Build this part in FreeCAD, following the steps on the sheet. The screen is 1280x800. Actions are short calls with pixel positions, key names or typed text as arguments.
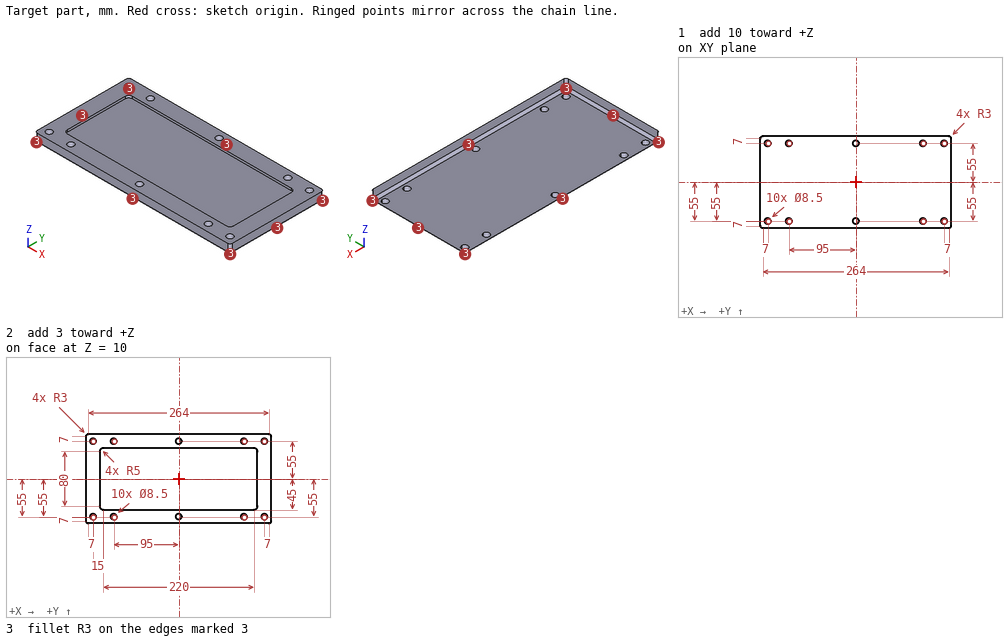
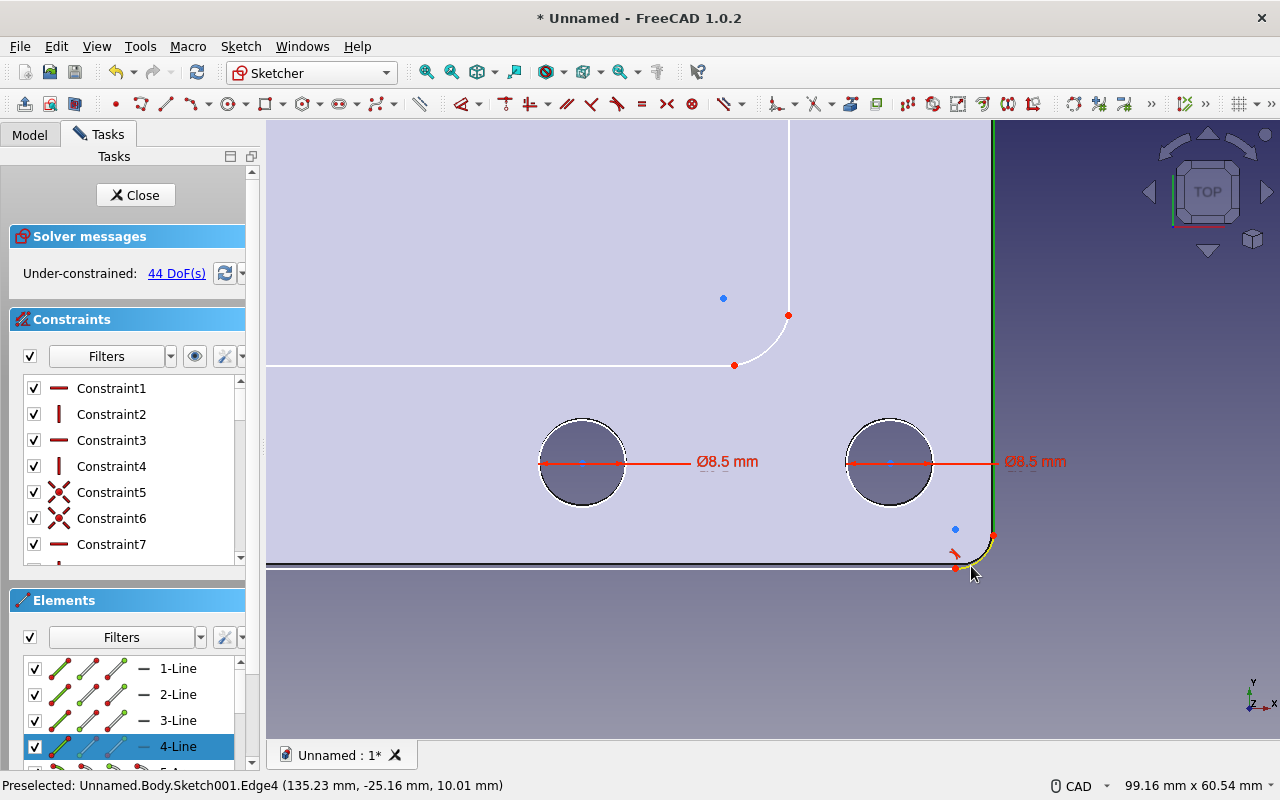
click(971, 565)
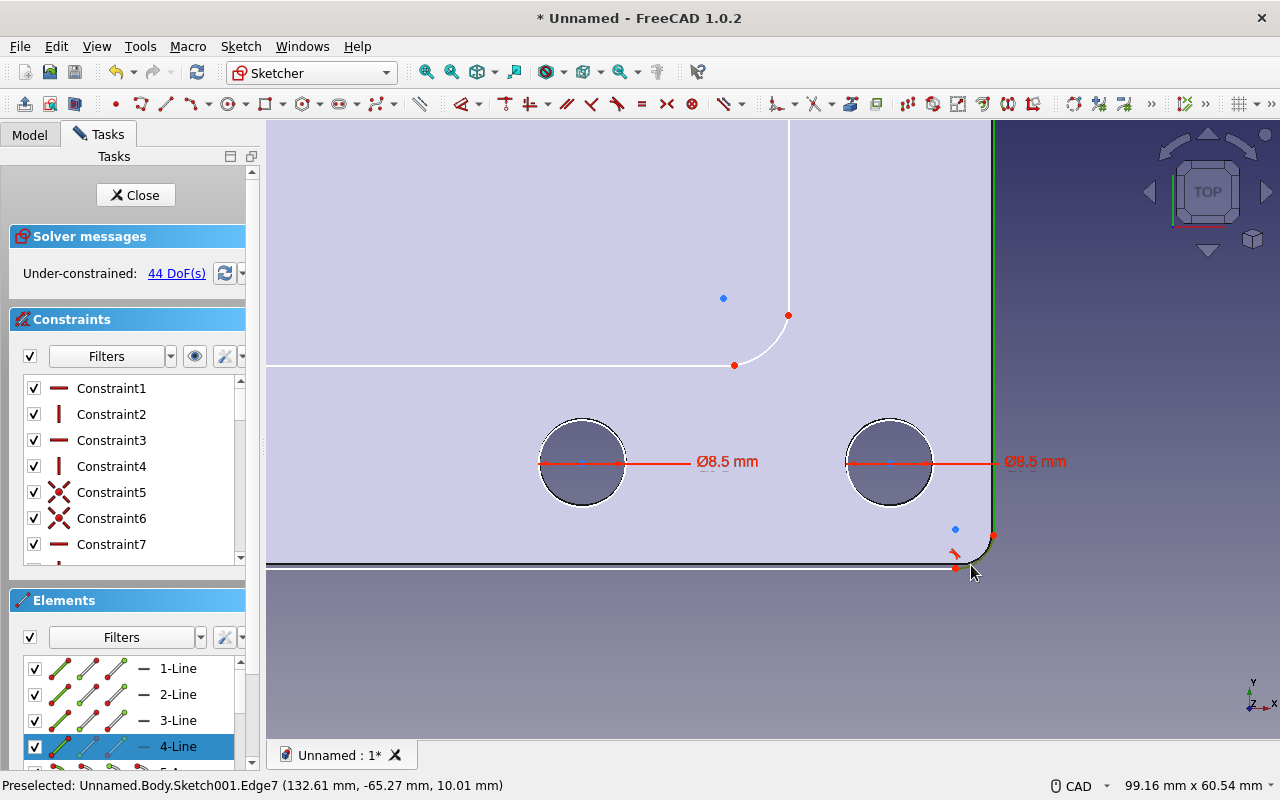
click(617, 104)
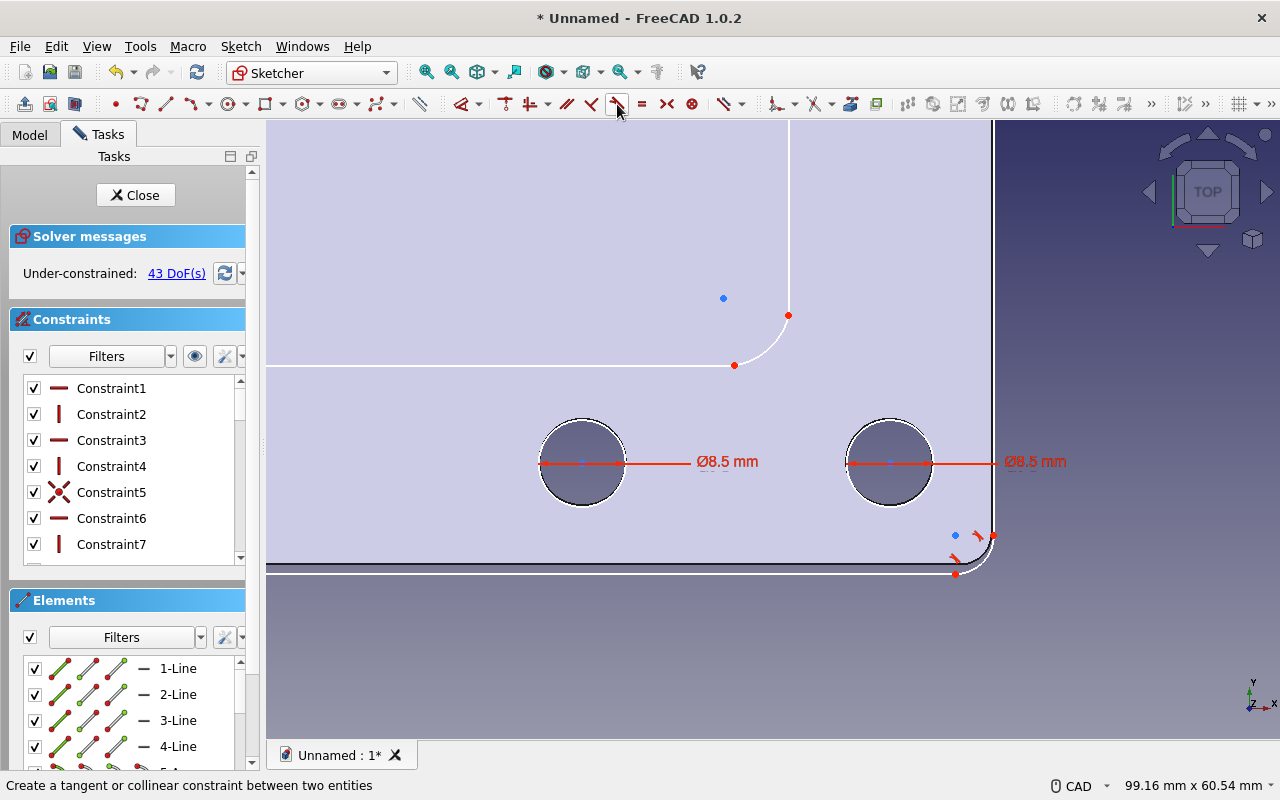
scroll(981, 564, down, 8)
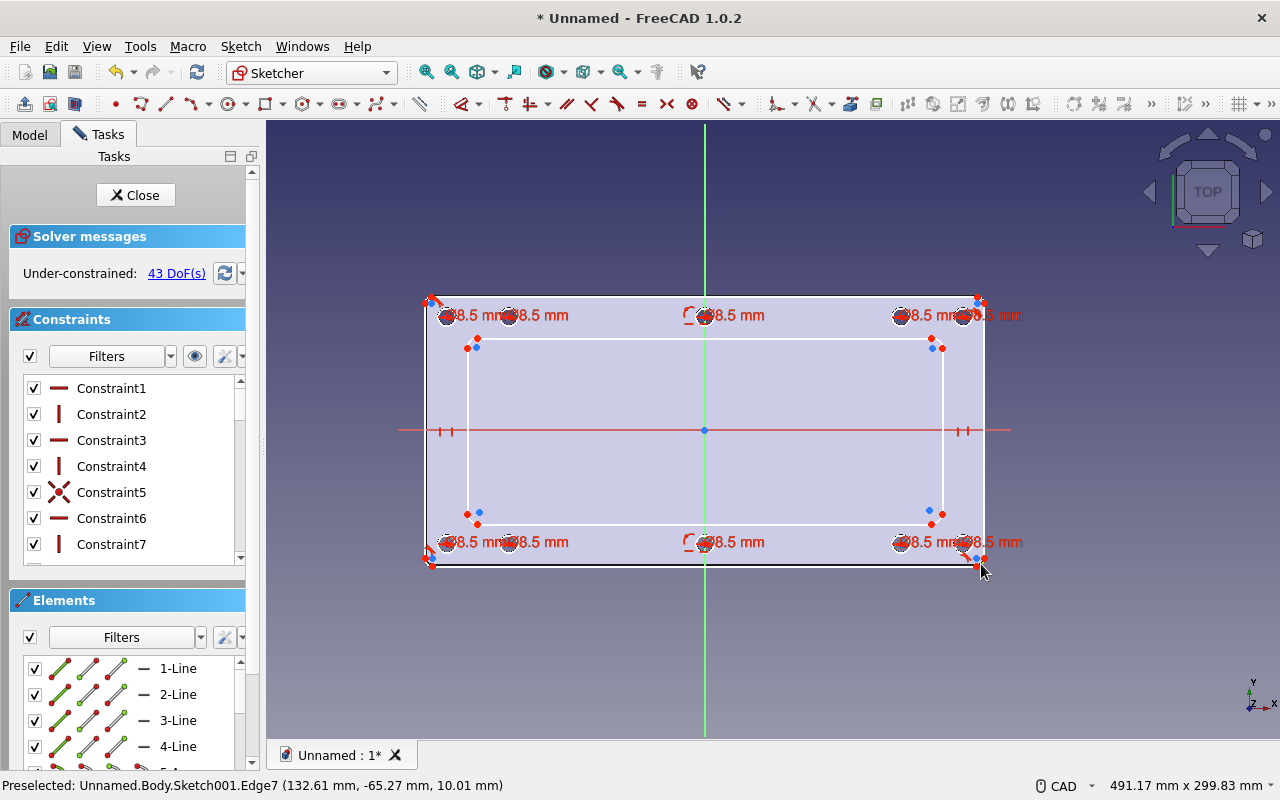
click(984, 482)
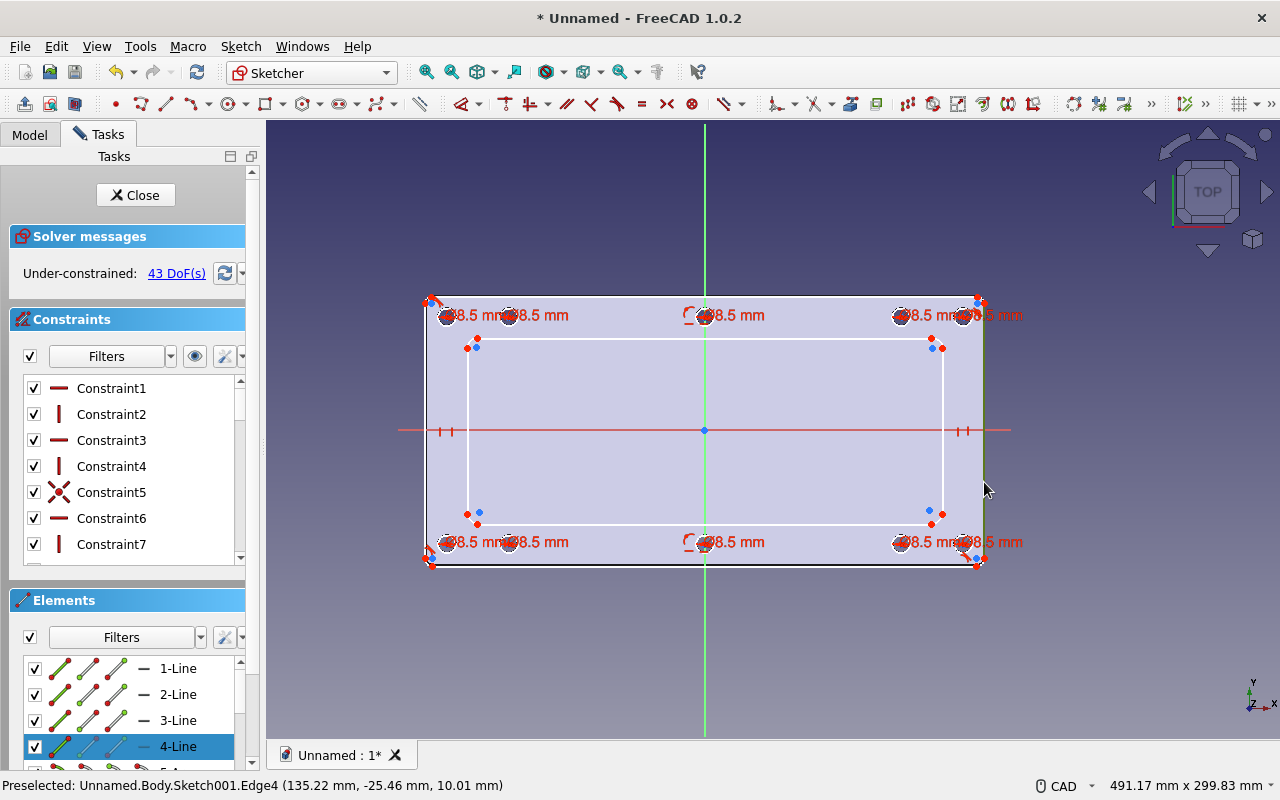
scroll(982, 299, up, 6)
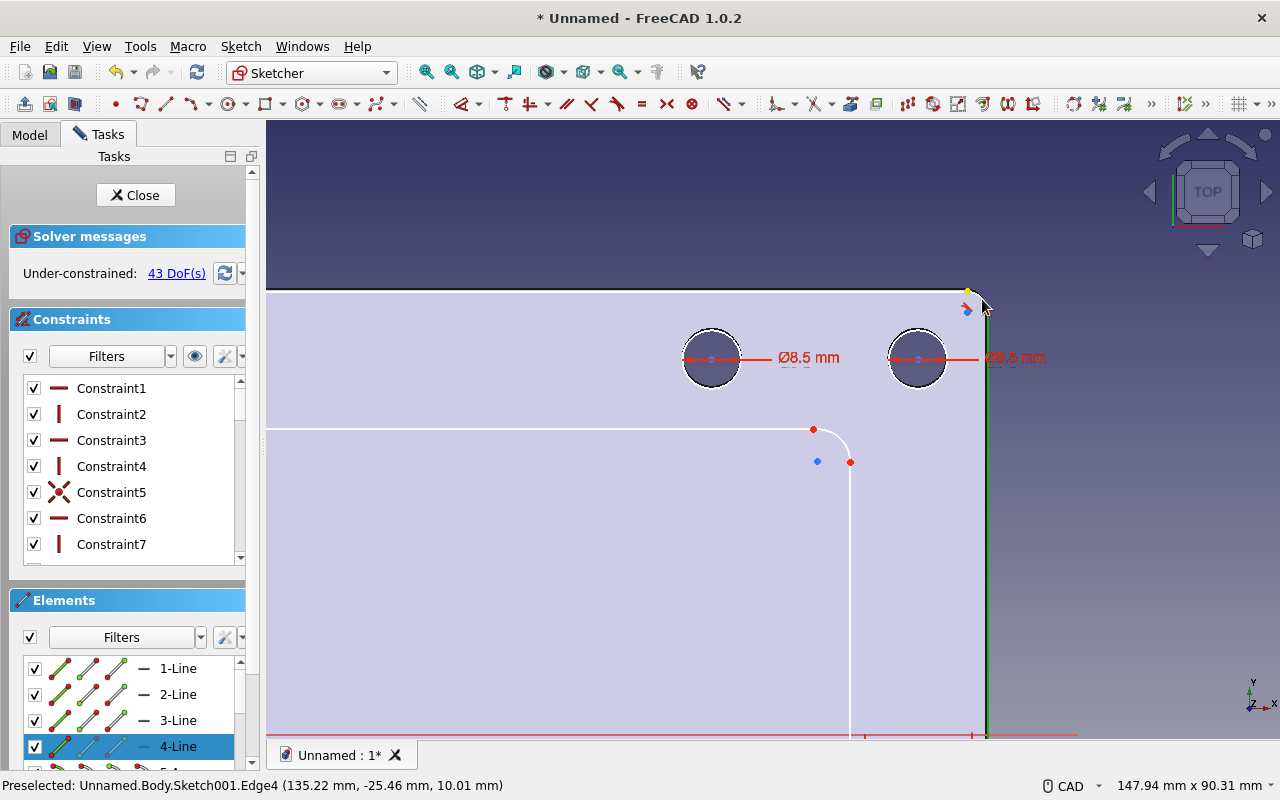
click(981, 298)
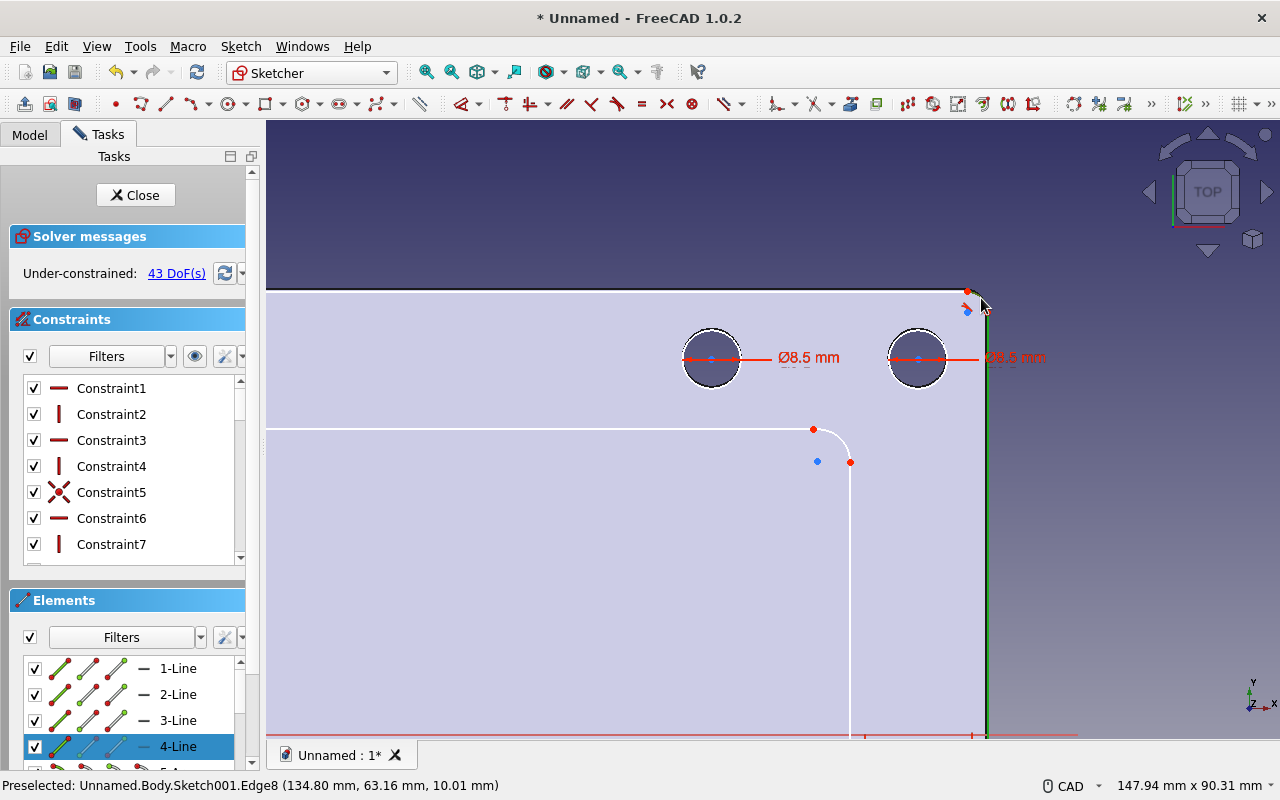
click(617, 104)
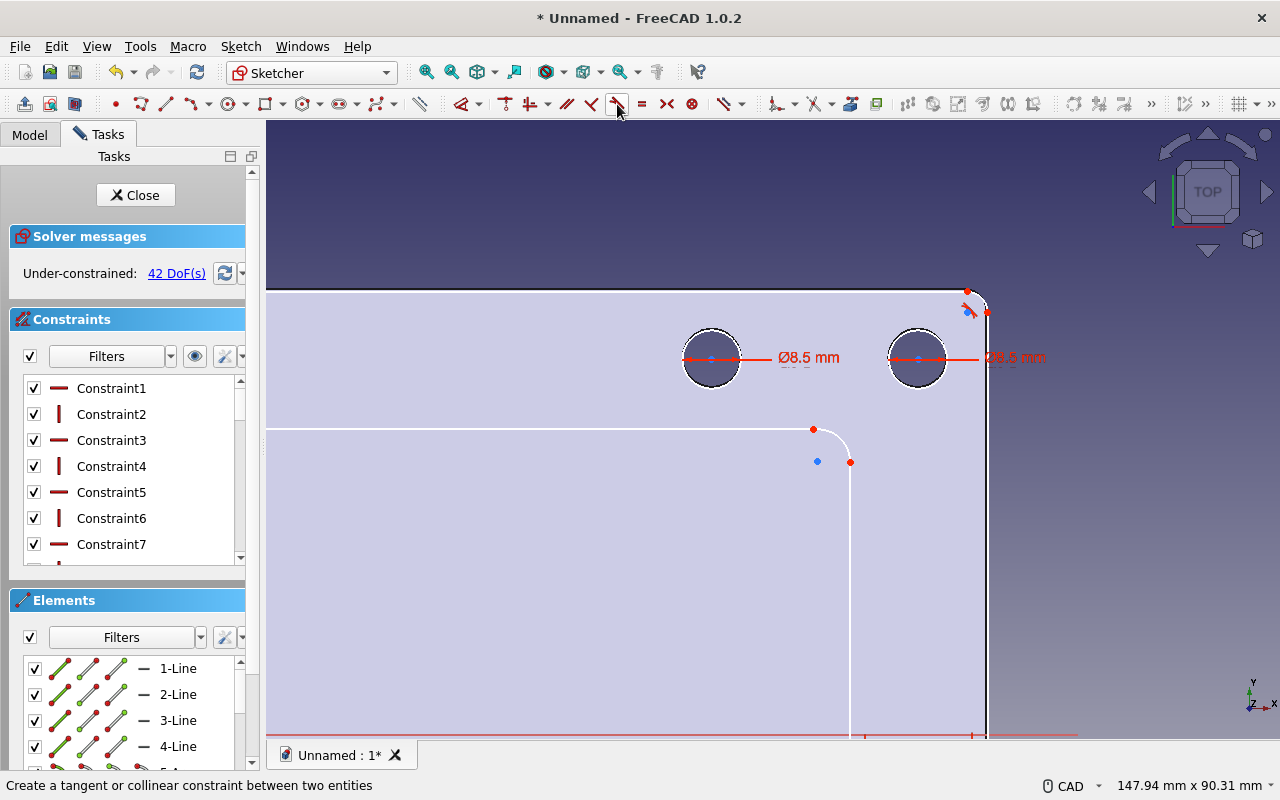
scroll(982, 298, down, 6)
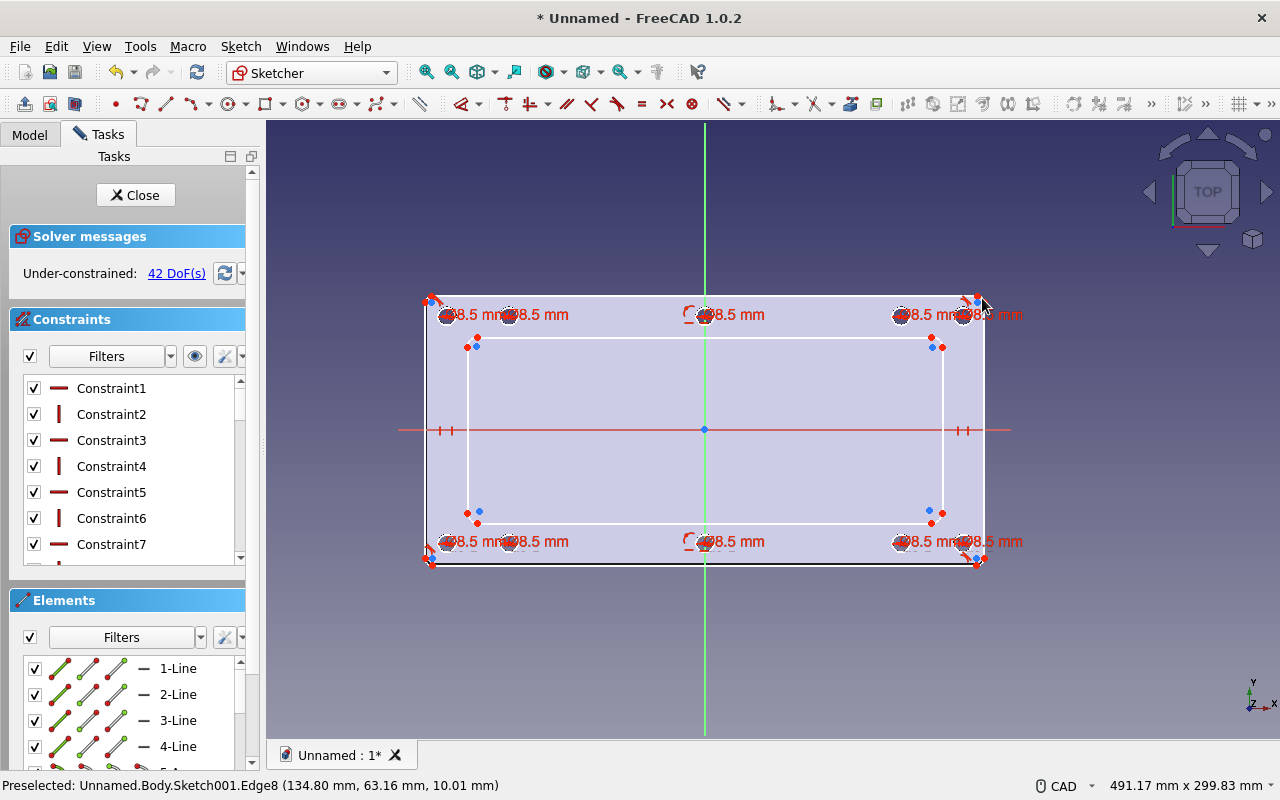
click(796, 524)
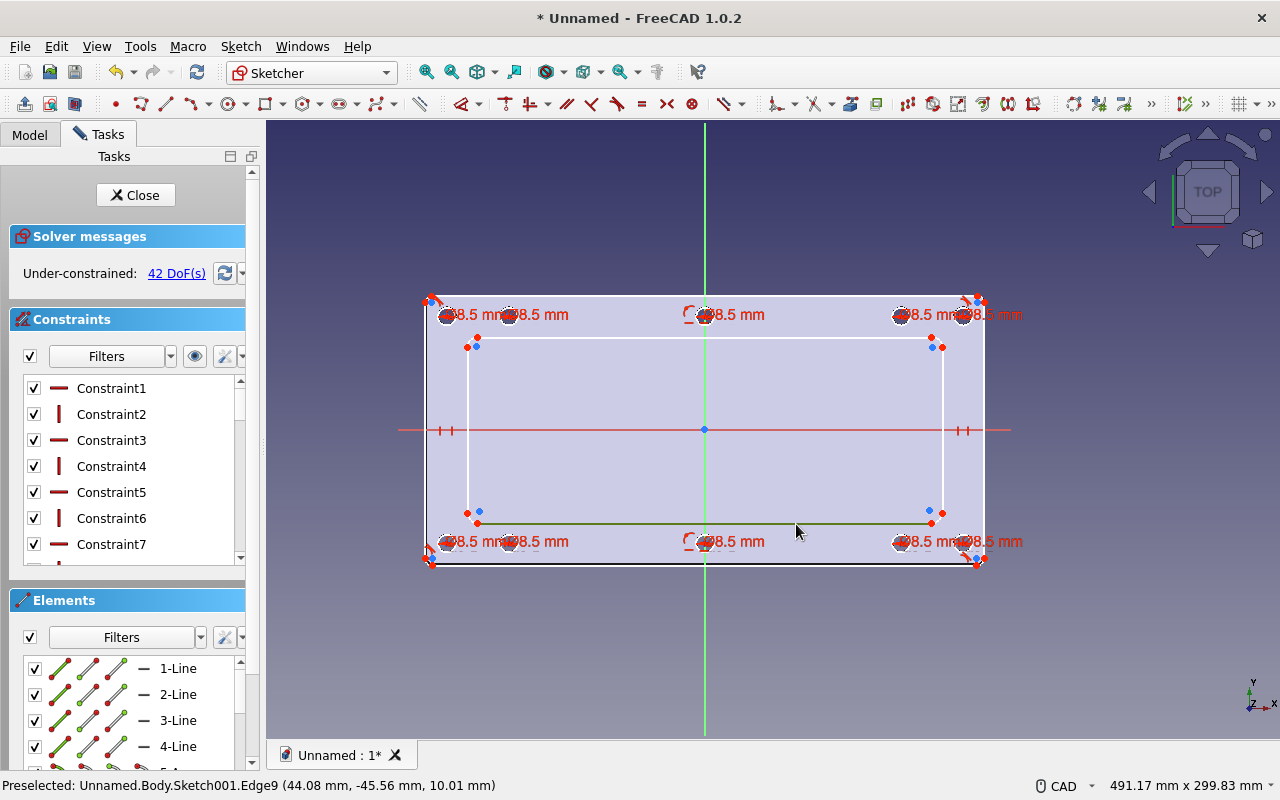
scroll(471, 520, up, 4)